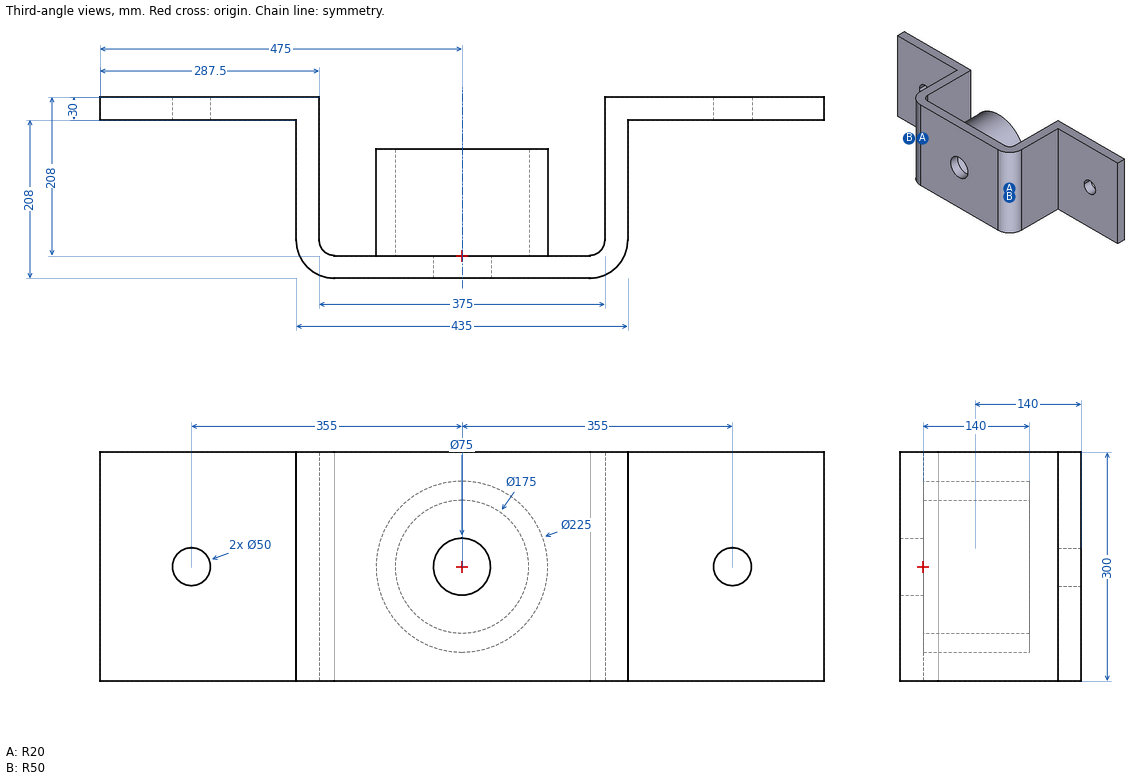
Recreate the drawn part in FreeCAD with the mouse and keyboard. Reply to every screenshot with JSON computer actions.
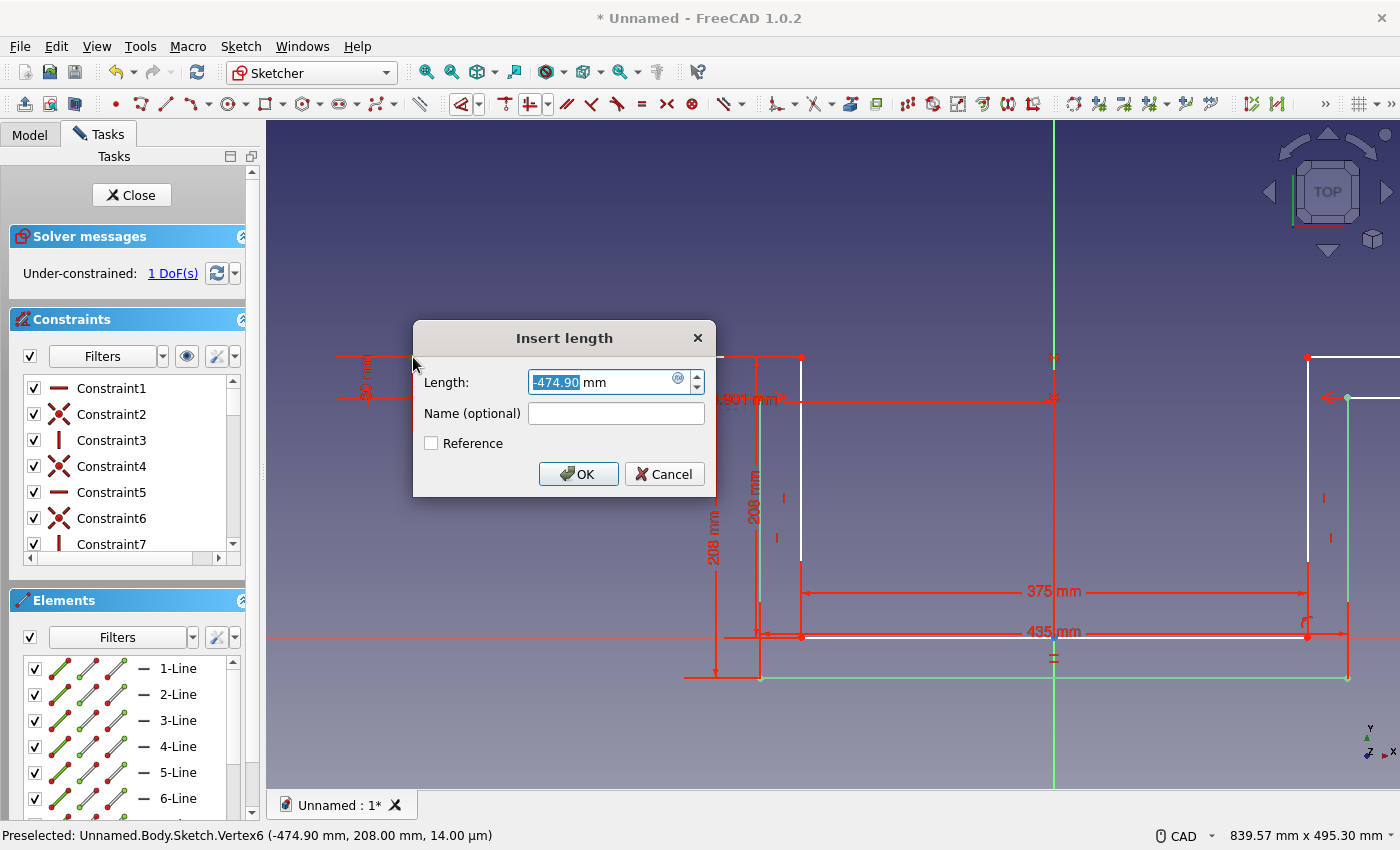
{"action": "type", "text": "-475"}
{"action": "key", "text": "Return"}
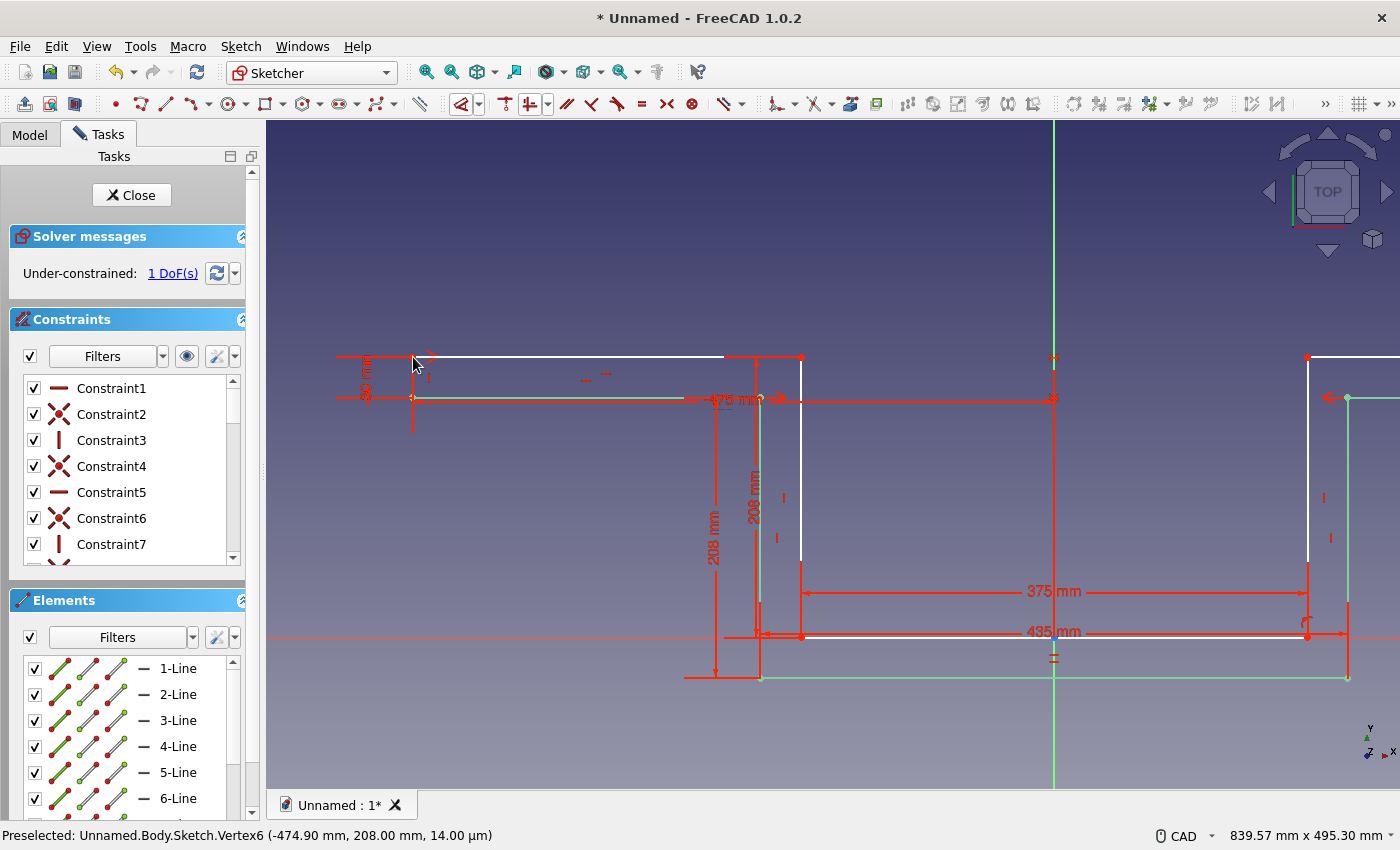
{"action": "left_click", "coordinate": [684, 357]}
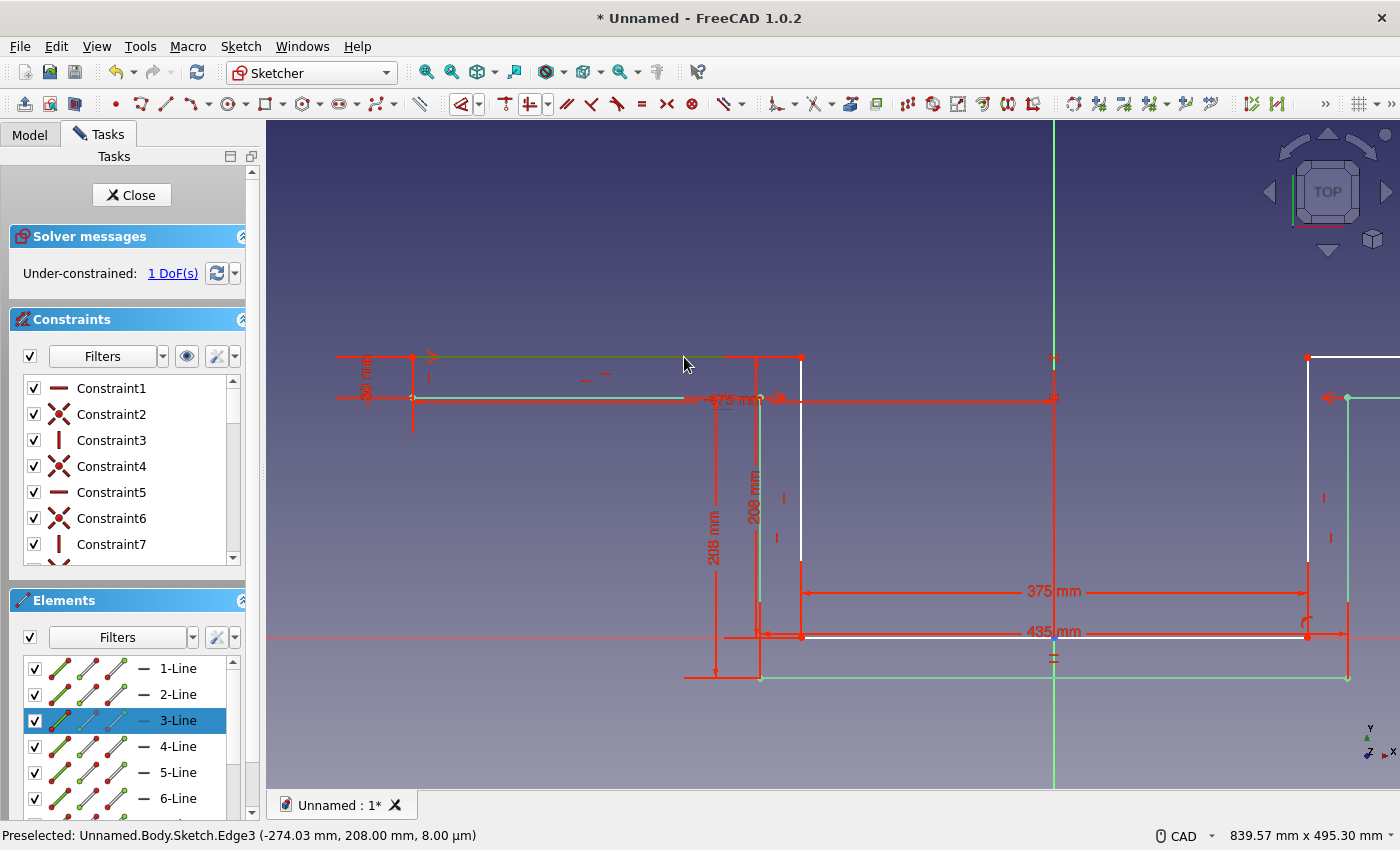
{"action": "left_click", "coordinate": [478, 104]}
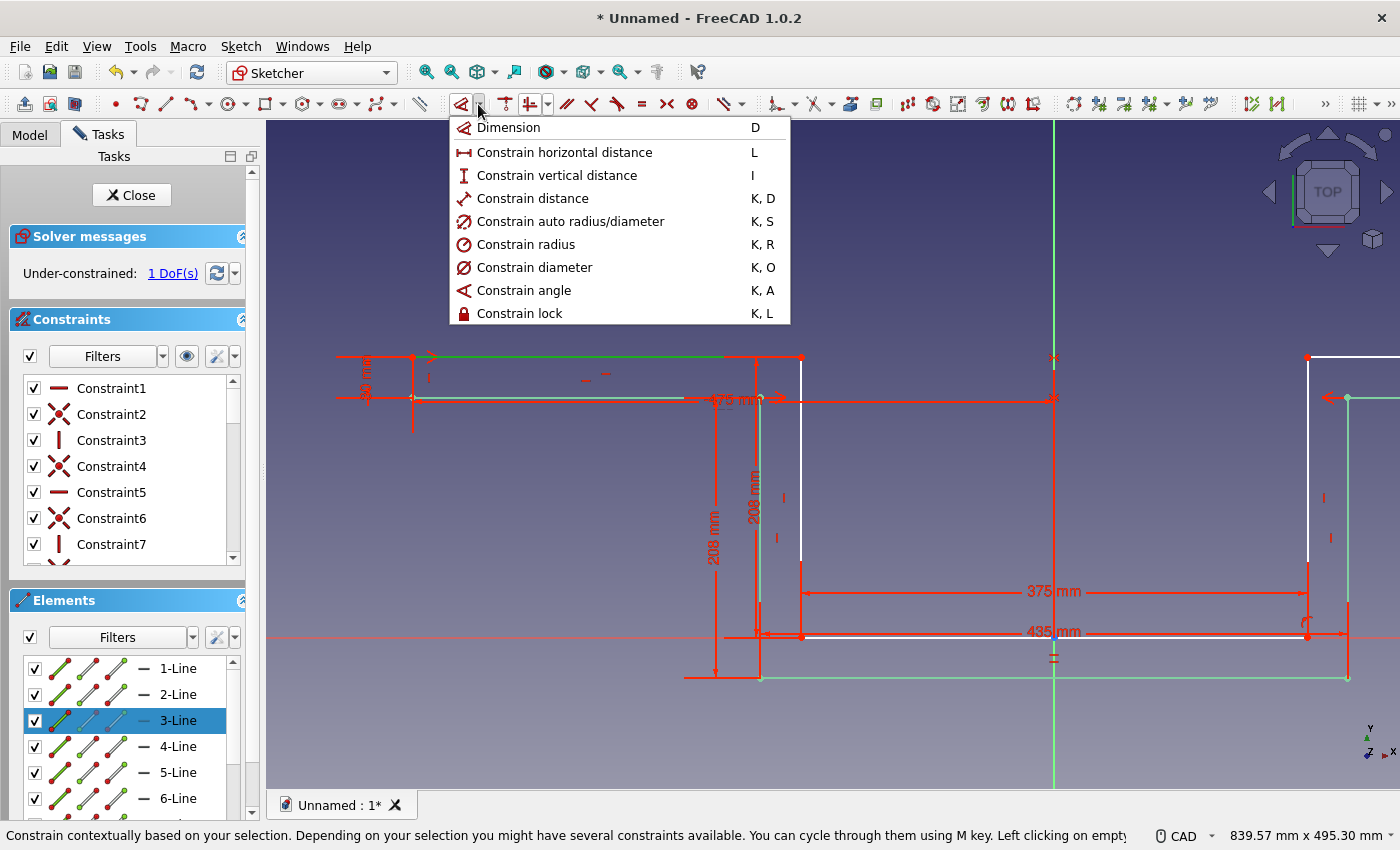
{"action": "left_click", "coordinate": [620, 152]}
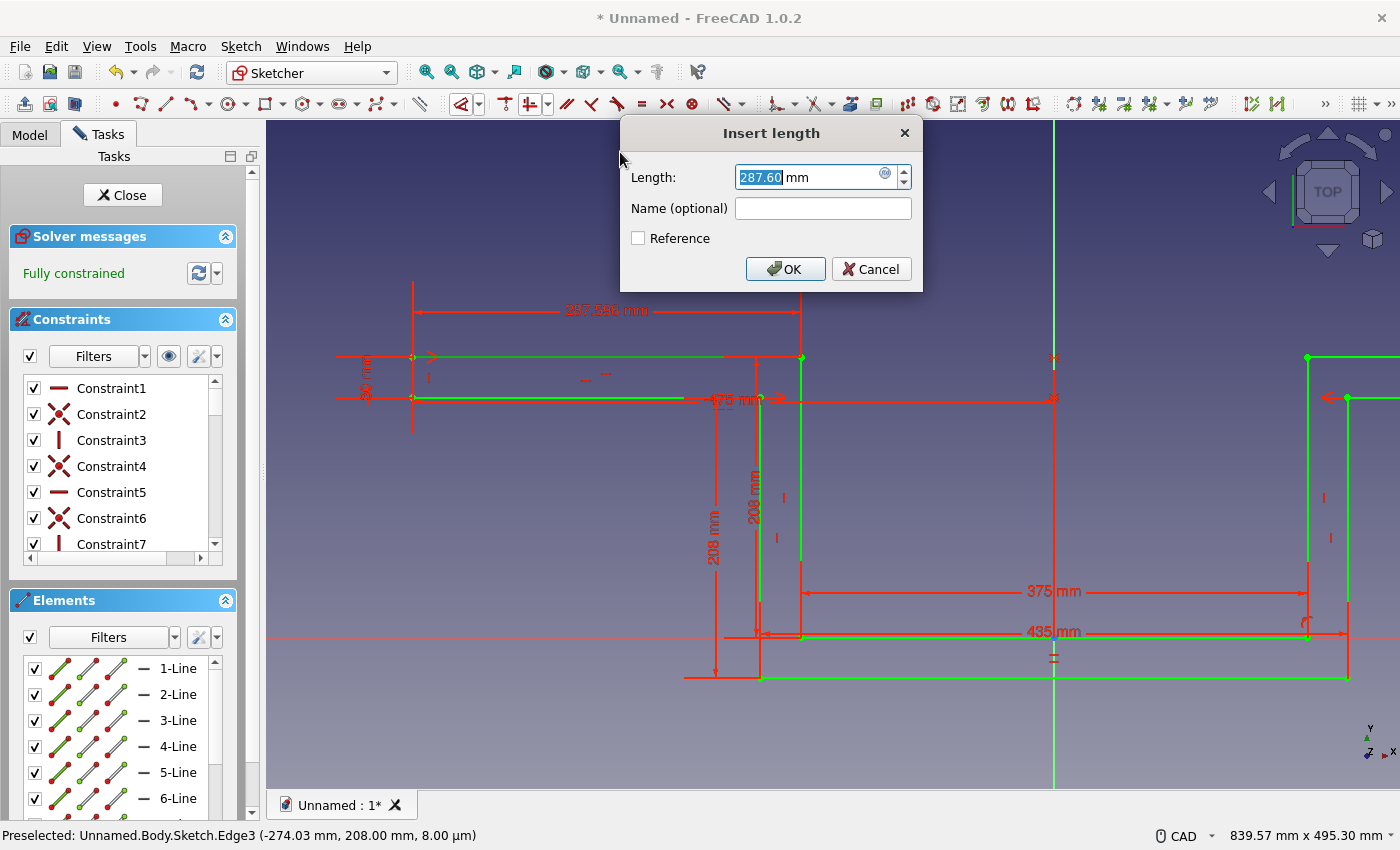
{"action": "type", "text": "287.5"}
{"action": "key", "text": "Return"}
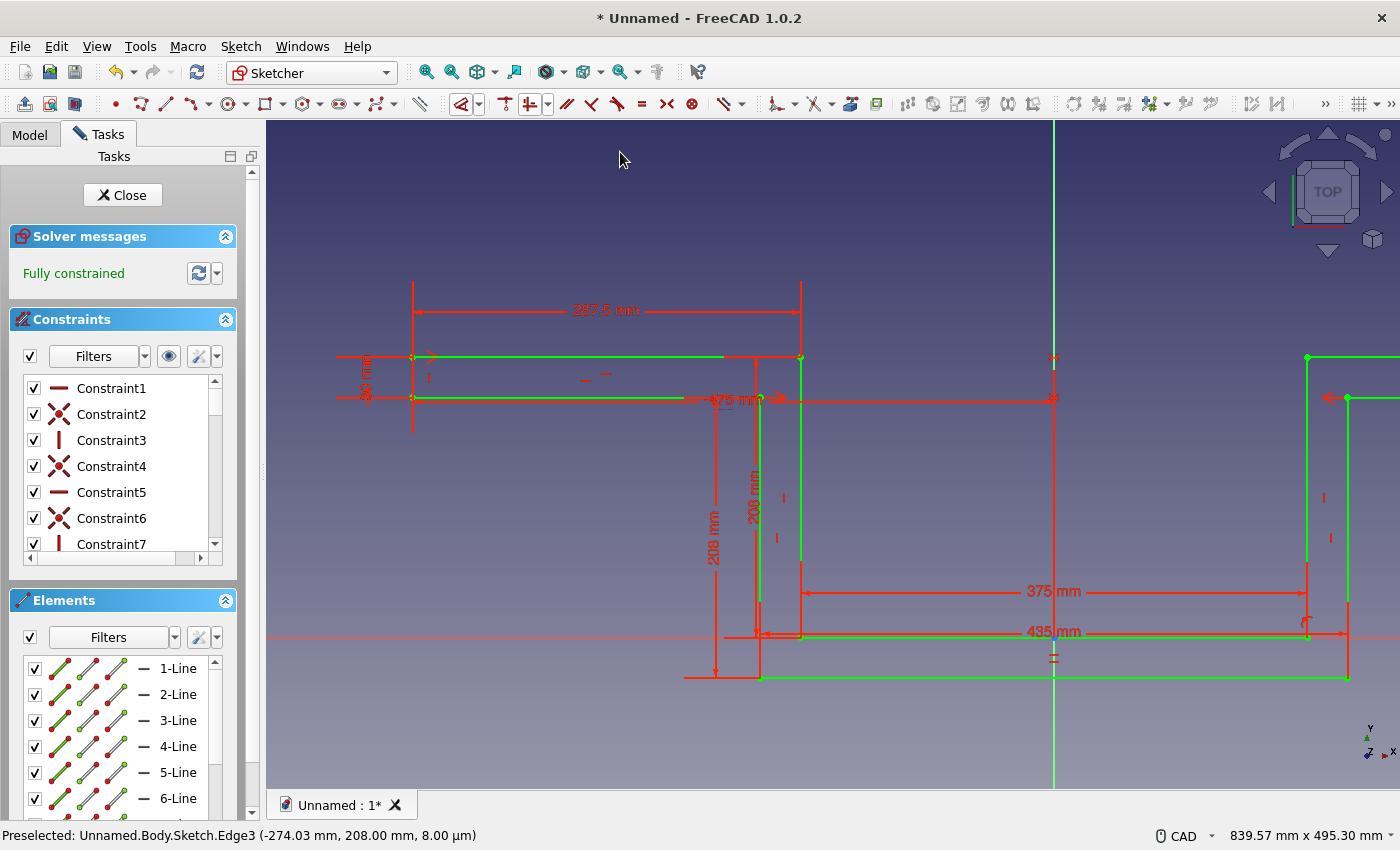
{"action": "left_click", "coordinate": [123, 195]}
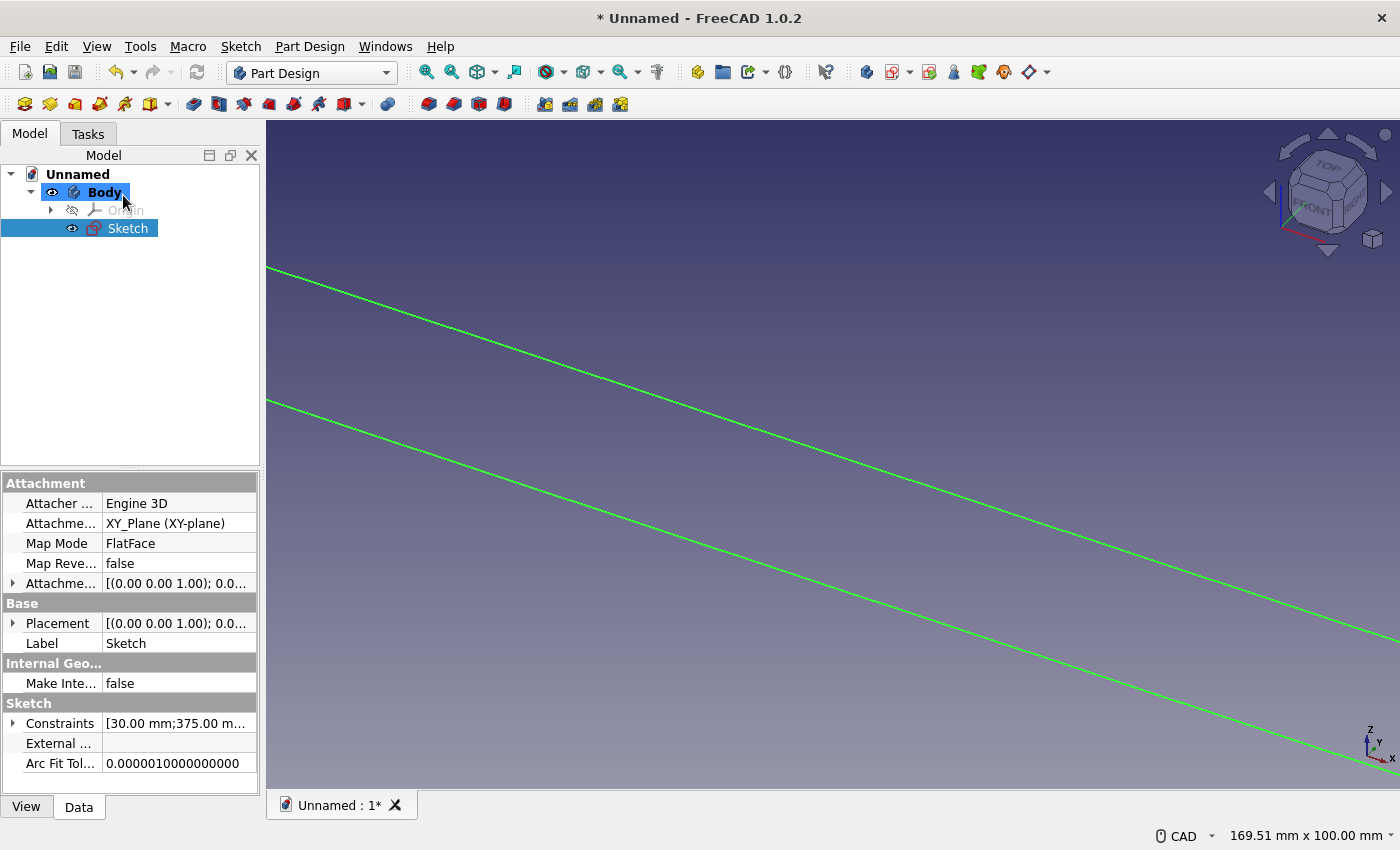
{"action": "left_click", "coordinate": [25, 104]}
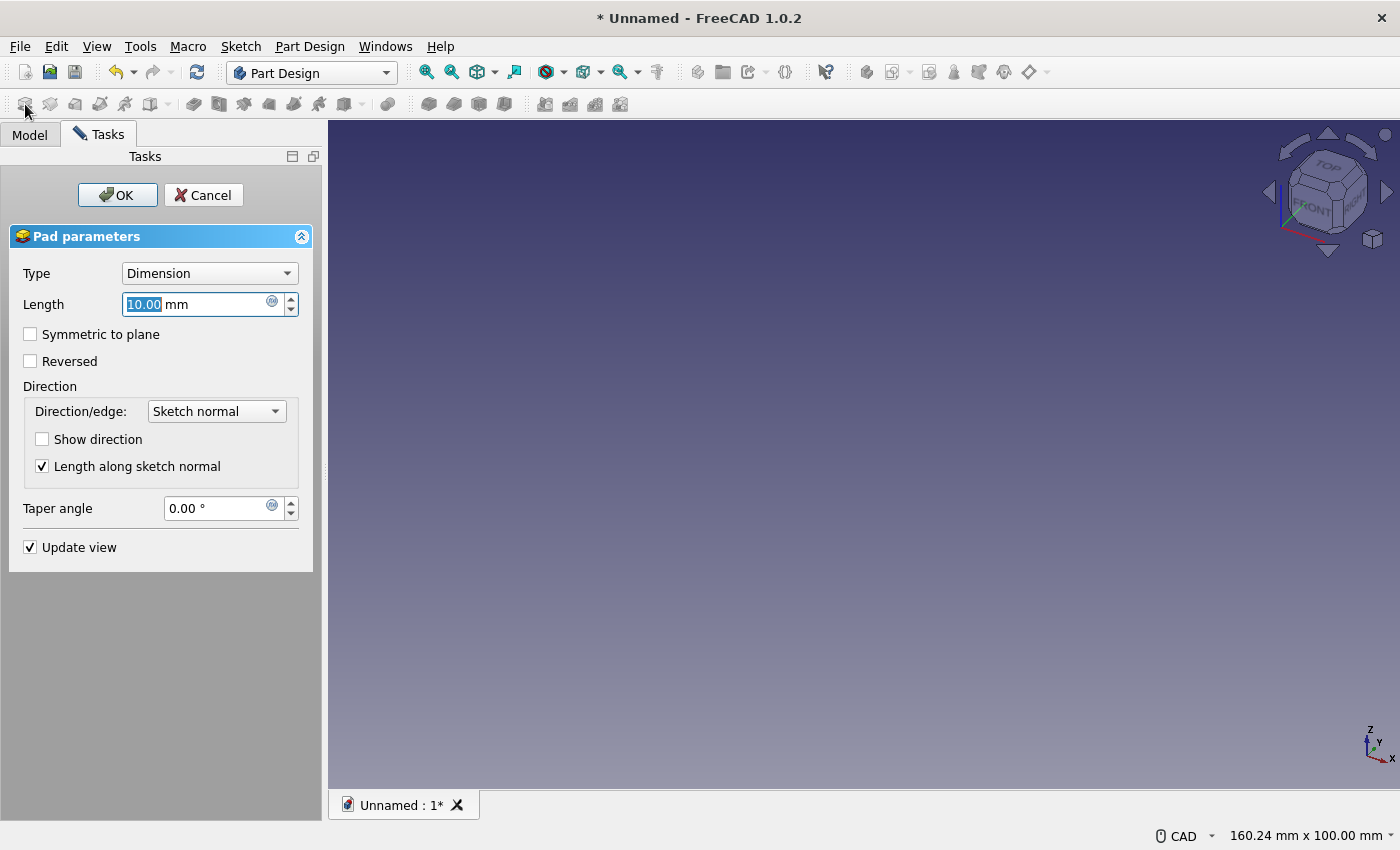
{"action": "type", "text": "300"}
{"action": "key", "text": "Tab"}